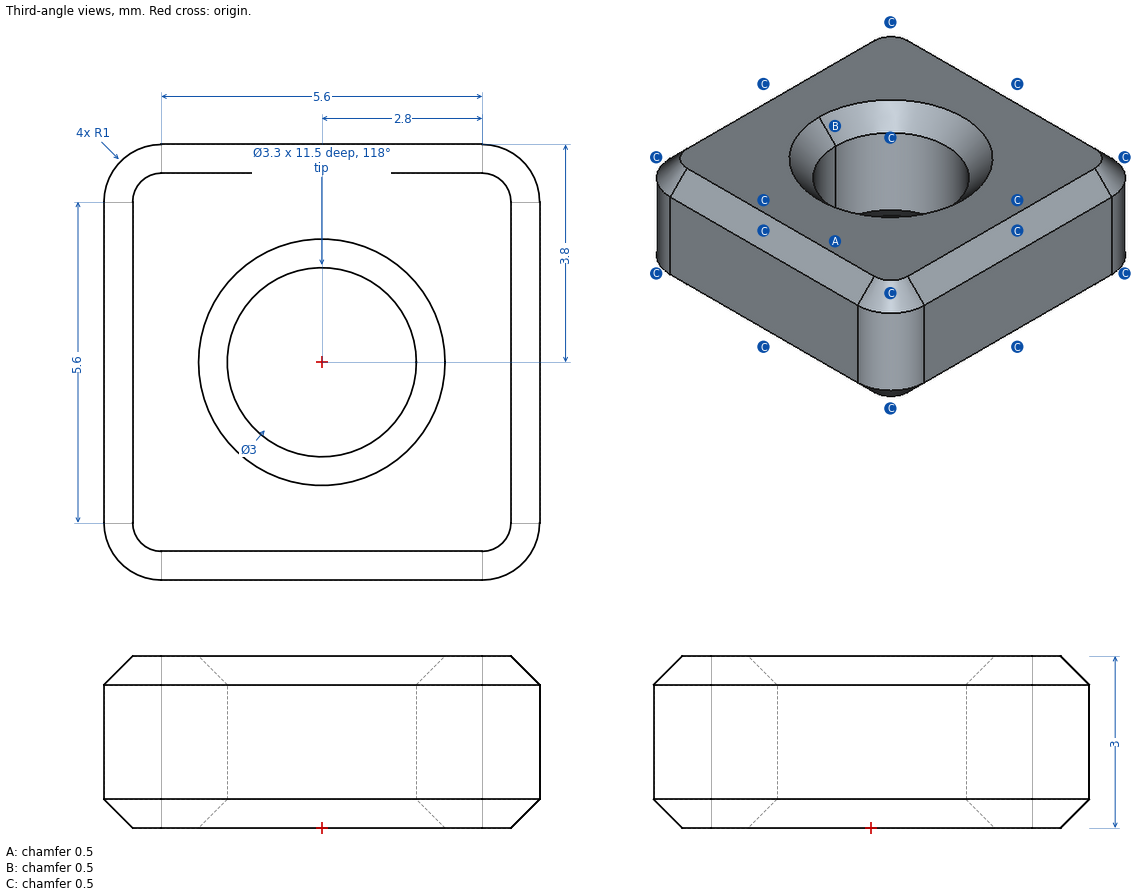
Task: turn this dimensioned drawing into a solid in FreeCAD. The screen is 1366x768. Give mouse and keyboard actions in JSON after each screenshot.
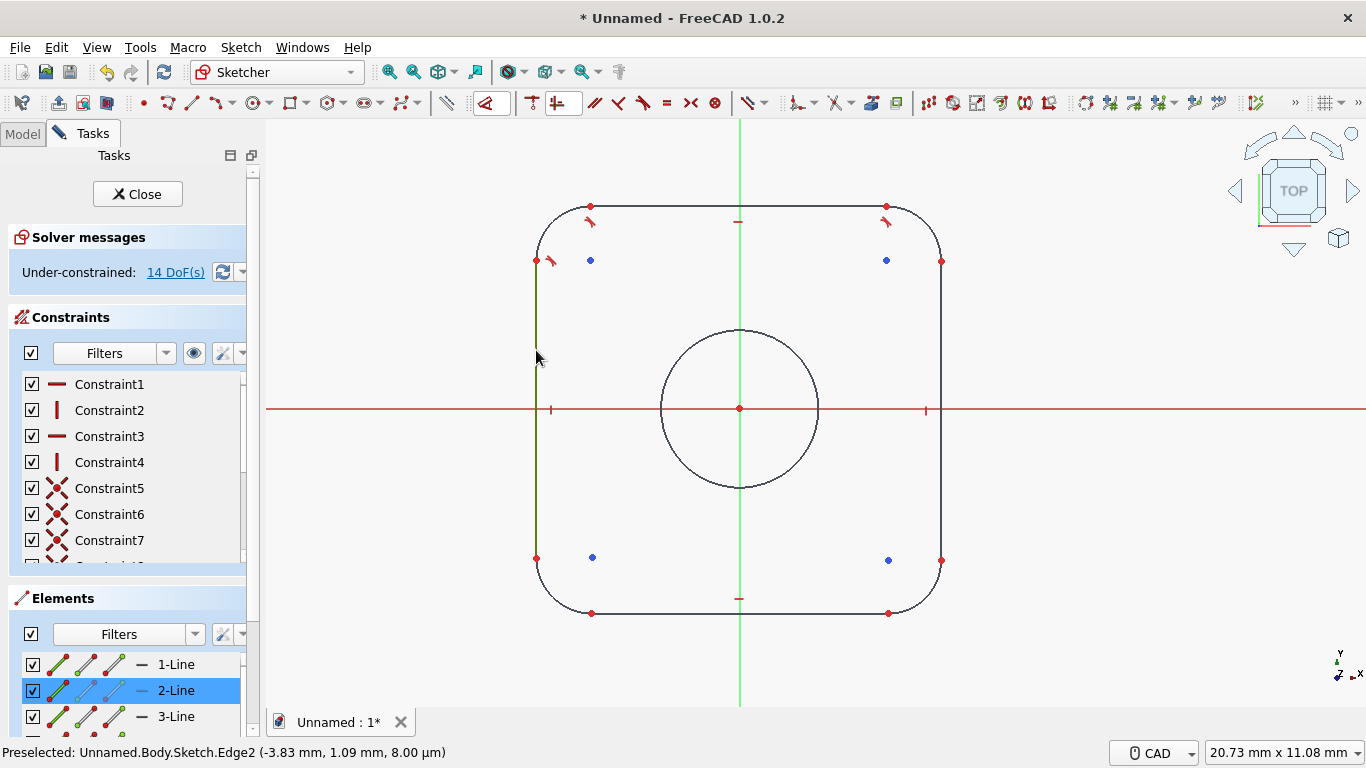
{"action": "left_click", "coordinate": [543, 583]}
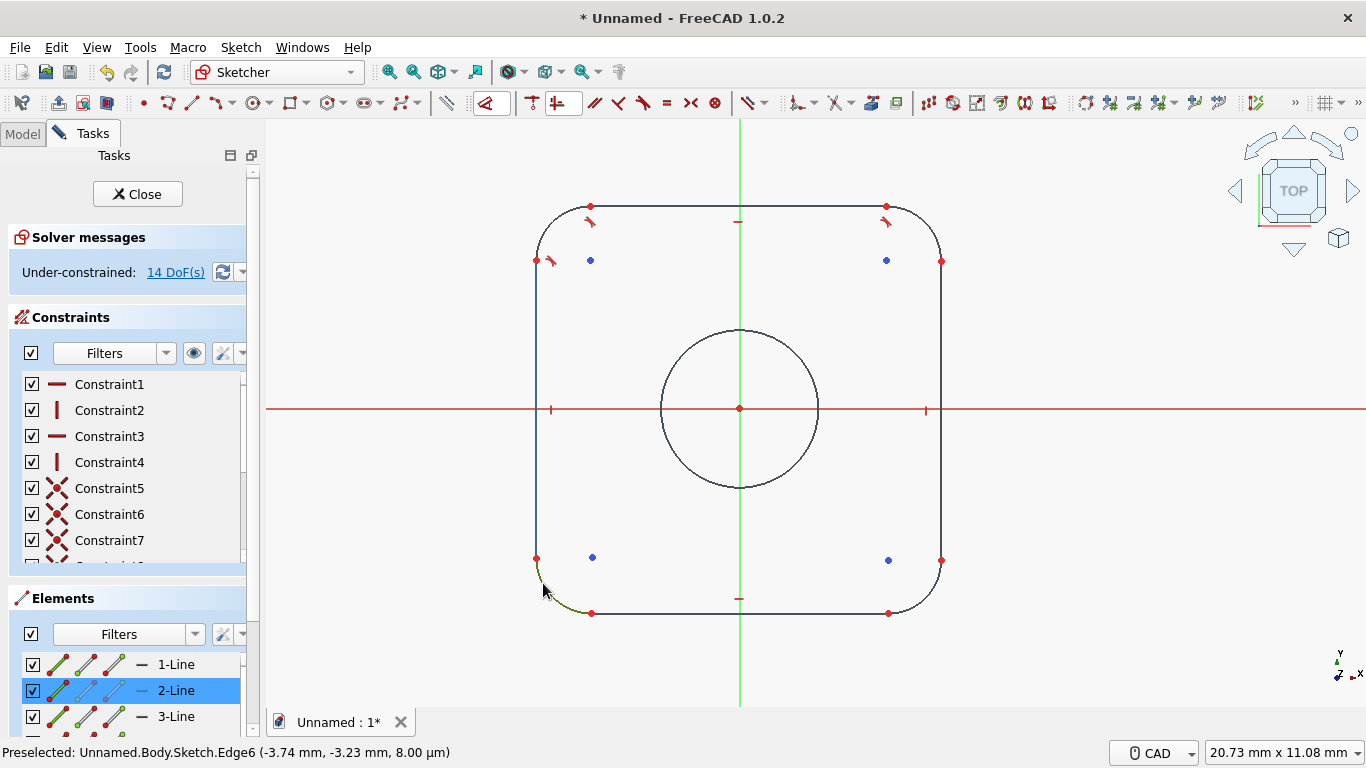
{"action": "key", "text": "t"}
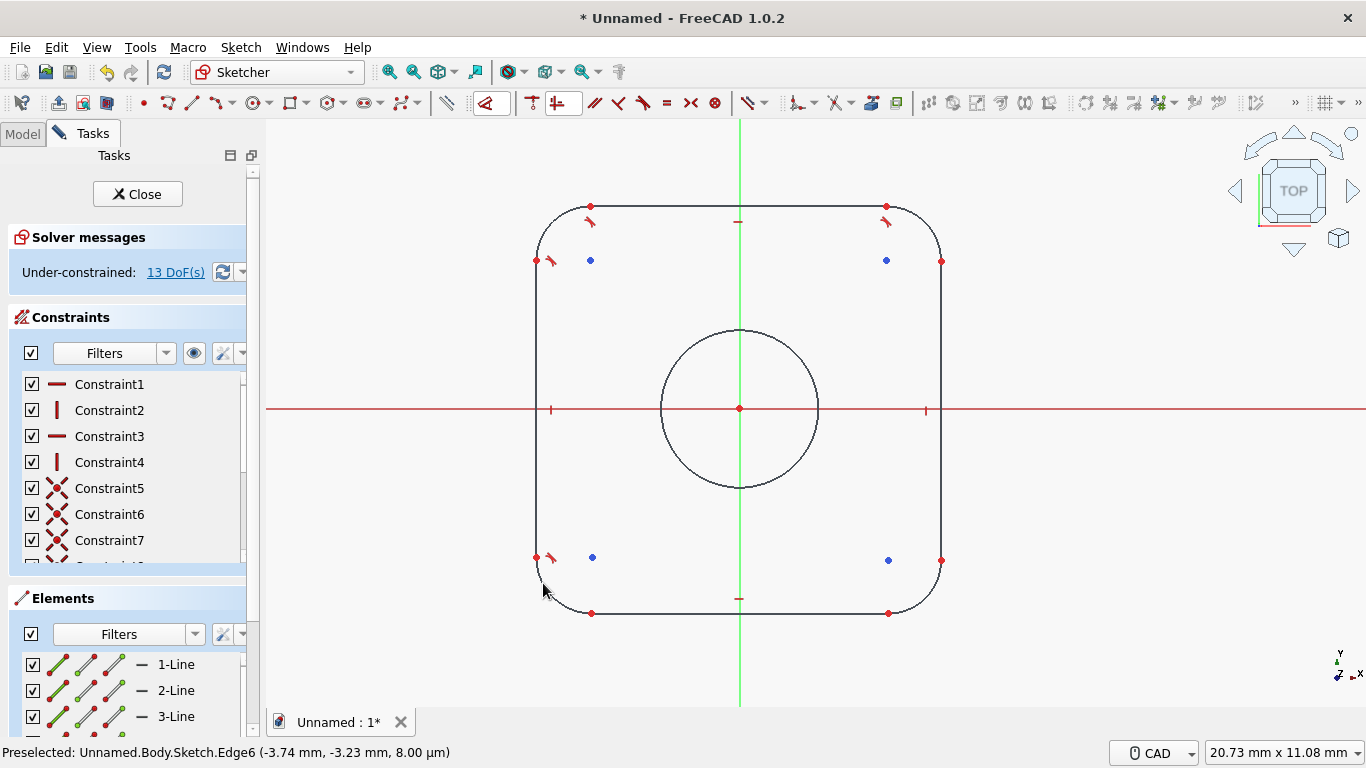
{"action": "left_click", "coordinate": [680, 614]}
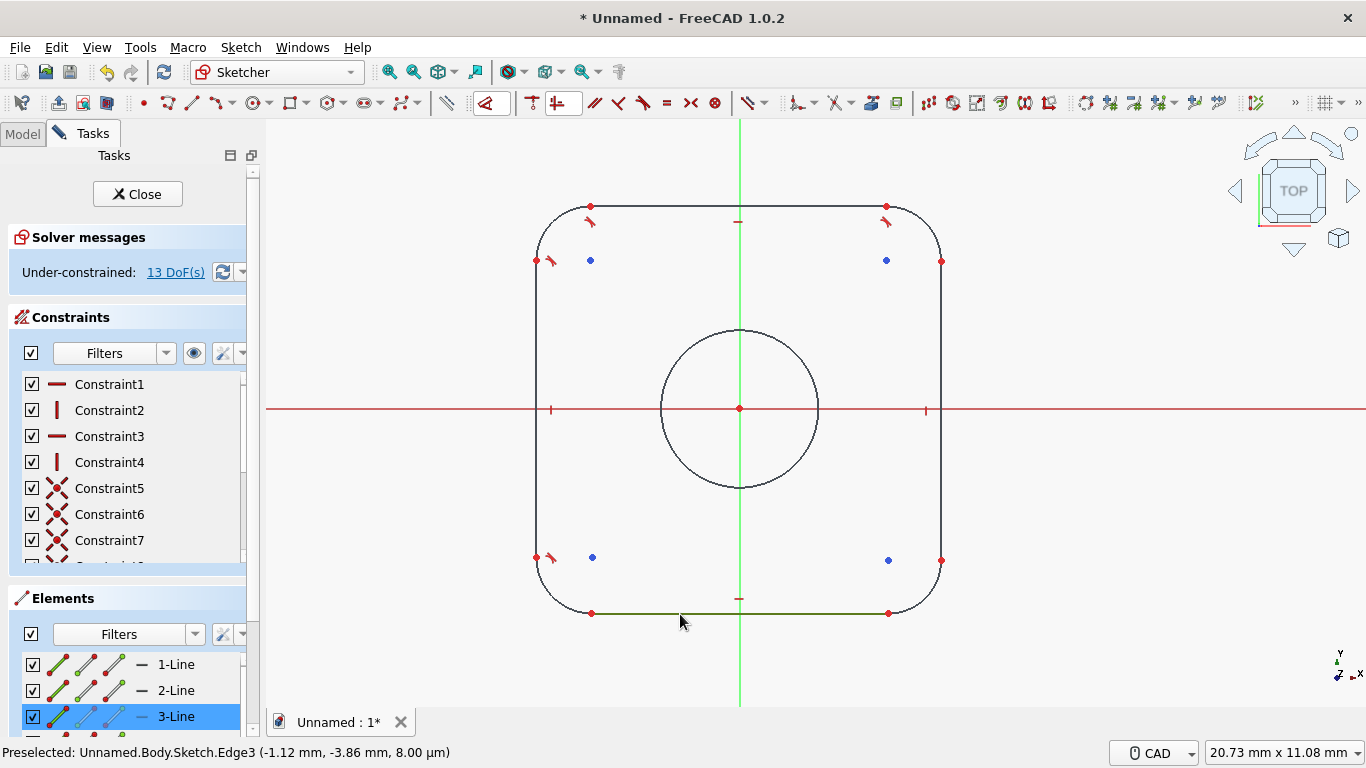
{"action": "left_click", "coordinate": [542, 582]}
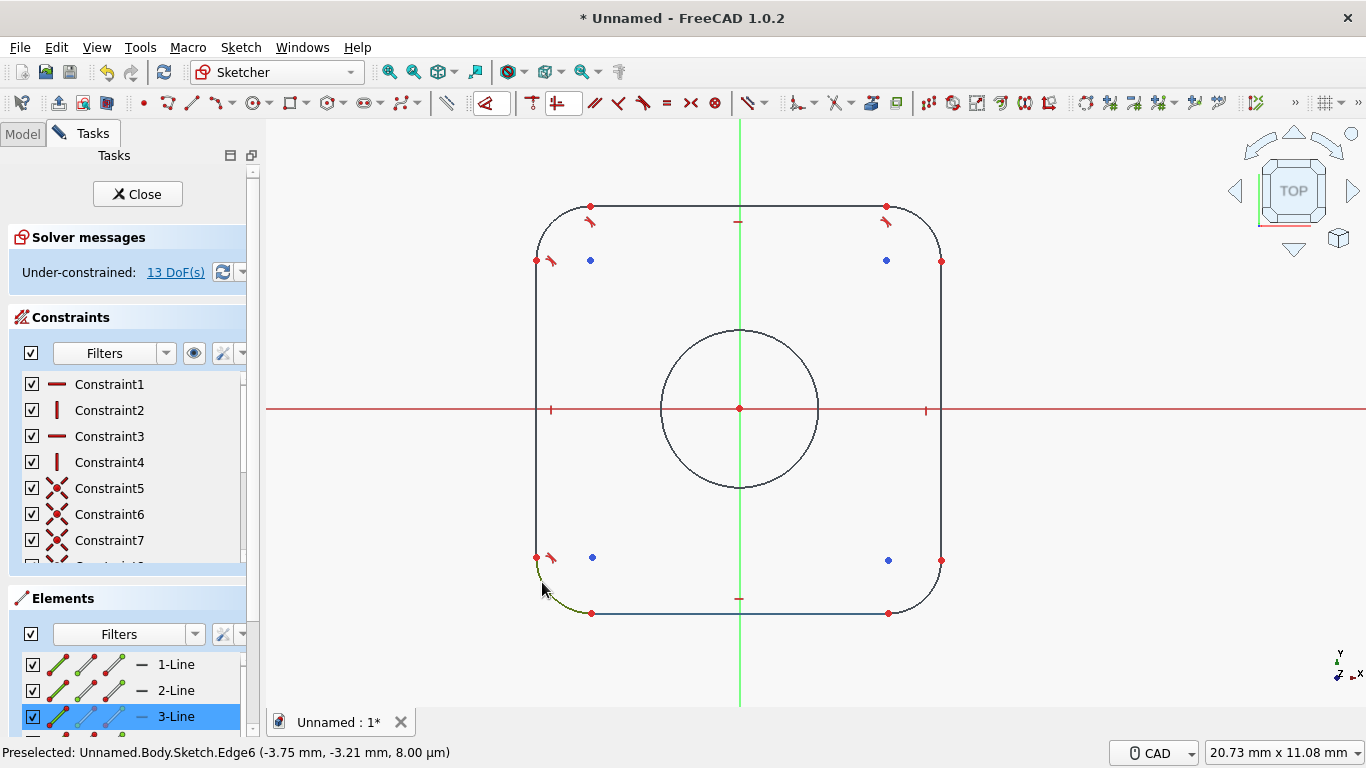
{"action": "key", "text": "t"}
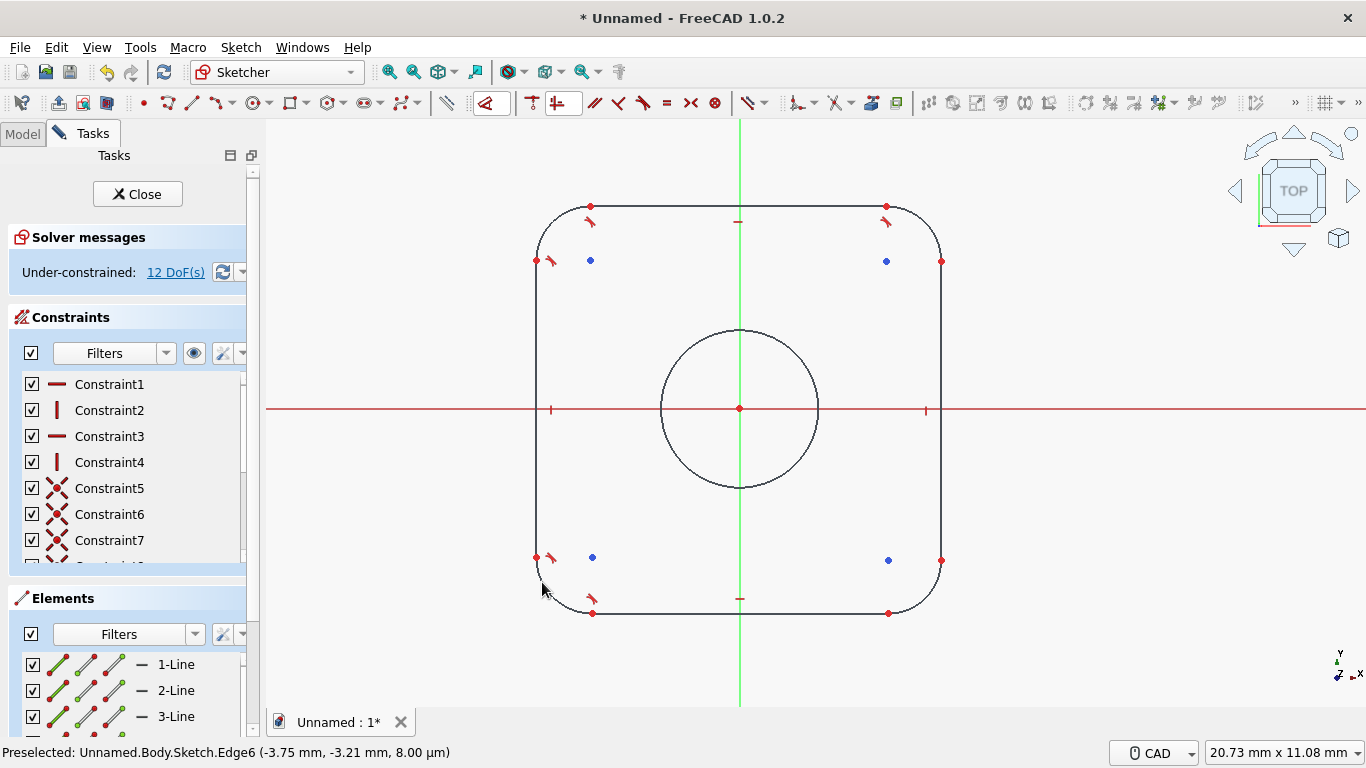
{"action": "left_click", "coordinate": [681, 614]}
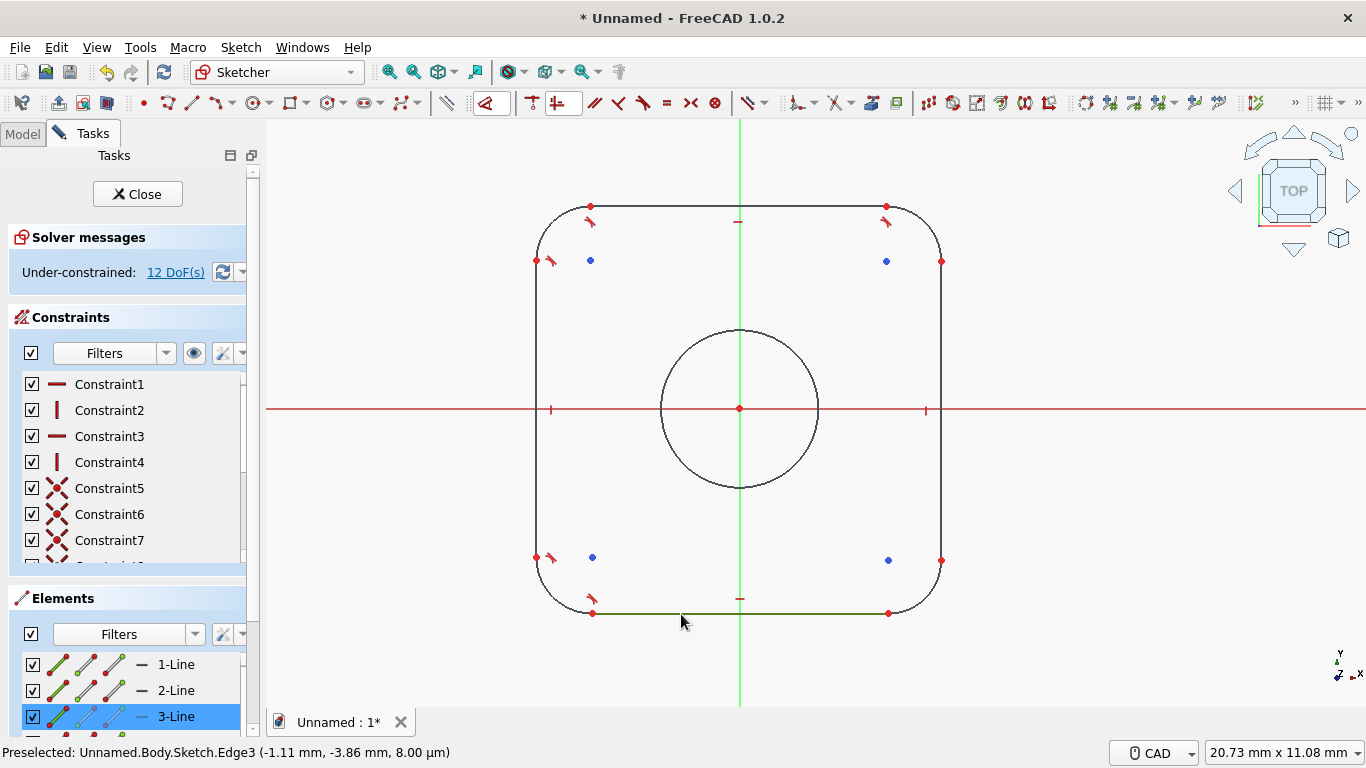
{"action": "left_click", "coordinate": [912, 608]}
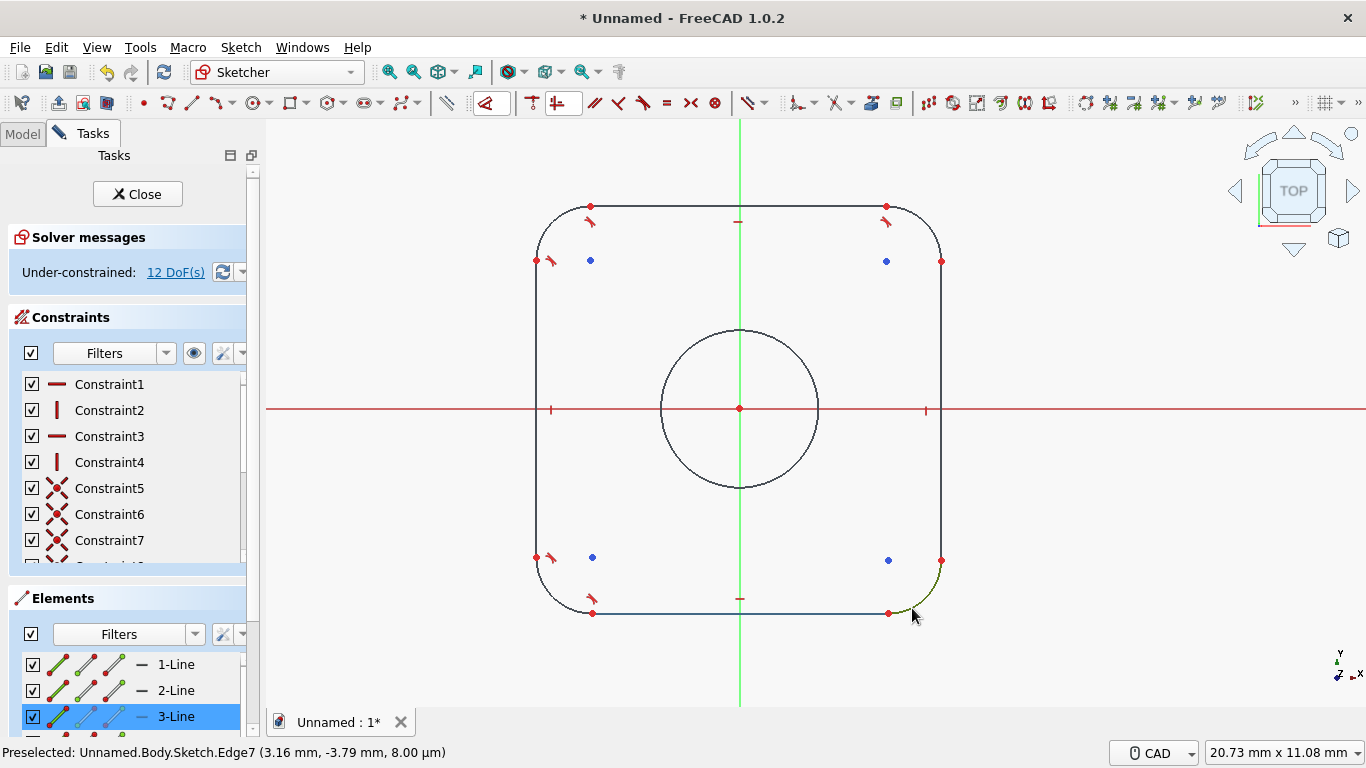
{"action": "key", "text": "t"}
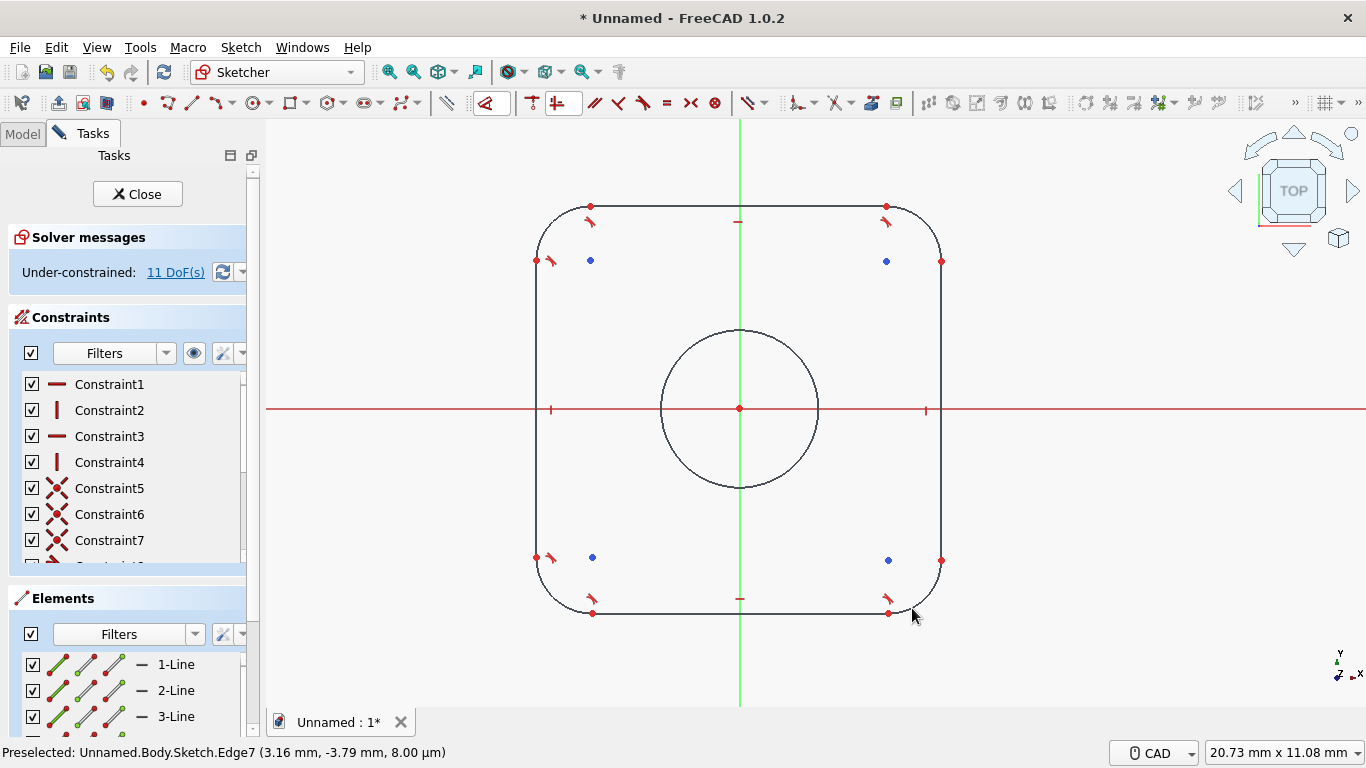
{"action": "left_click", "coordinate": [941, 471]}